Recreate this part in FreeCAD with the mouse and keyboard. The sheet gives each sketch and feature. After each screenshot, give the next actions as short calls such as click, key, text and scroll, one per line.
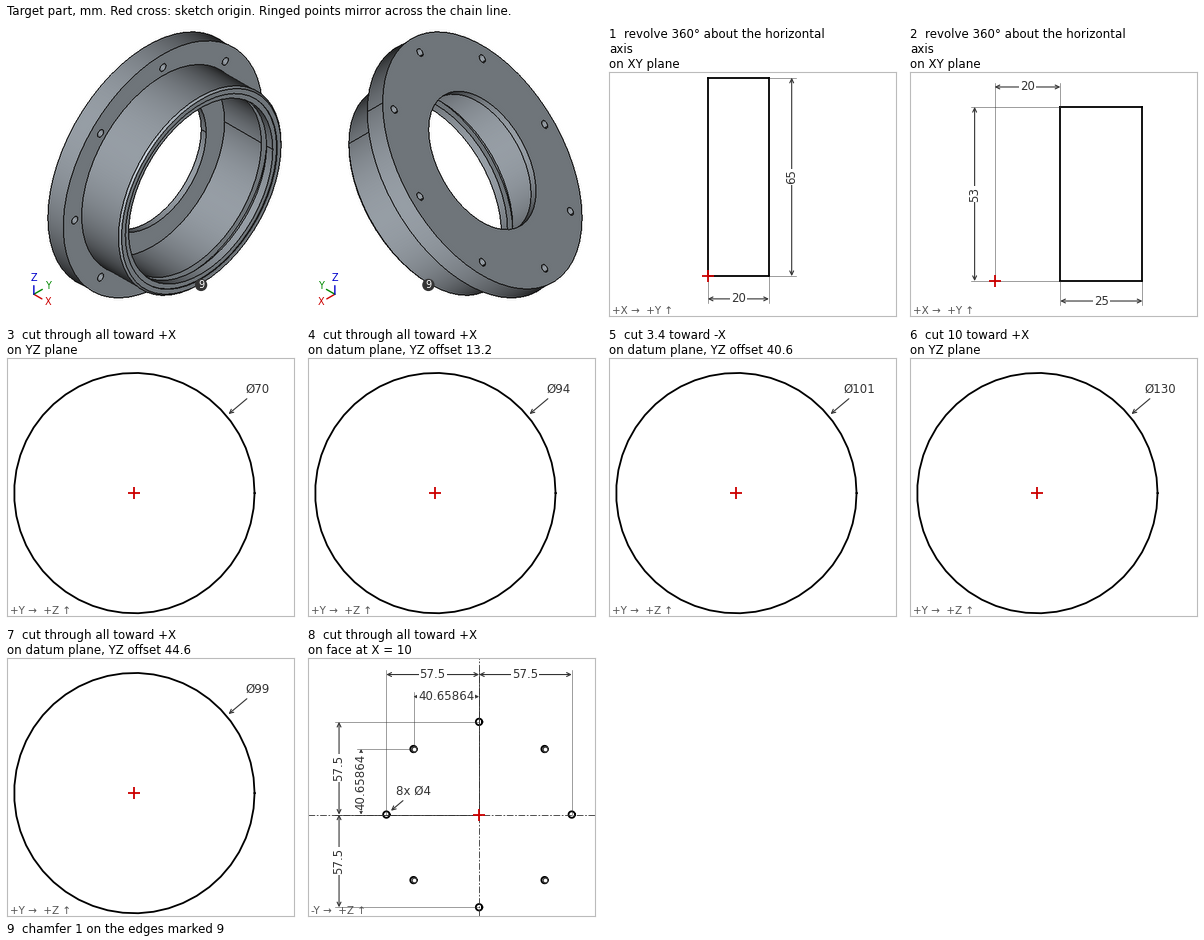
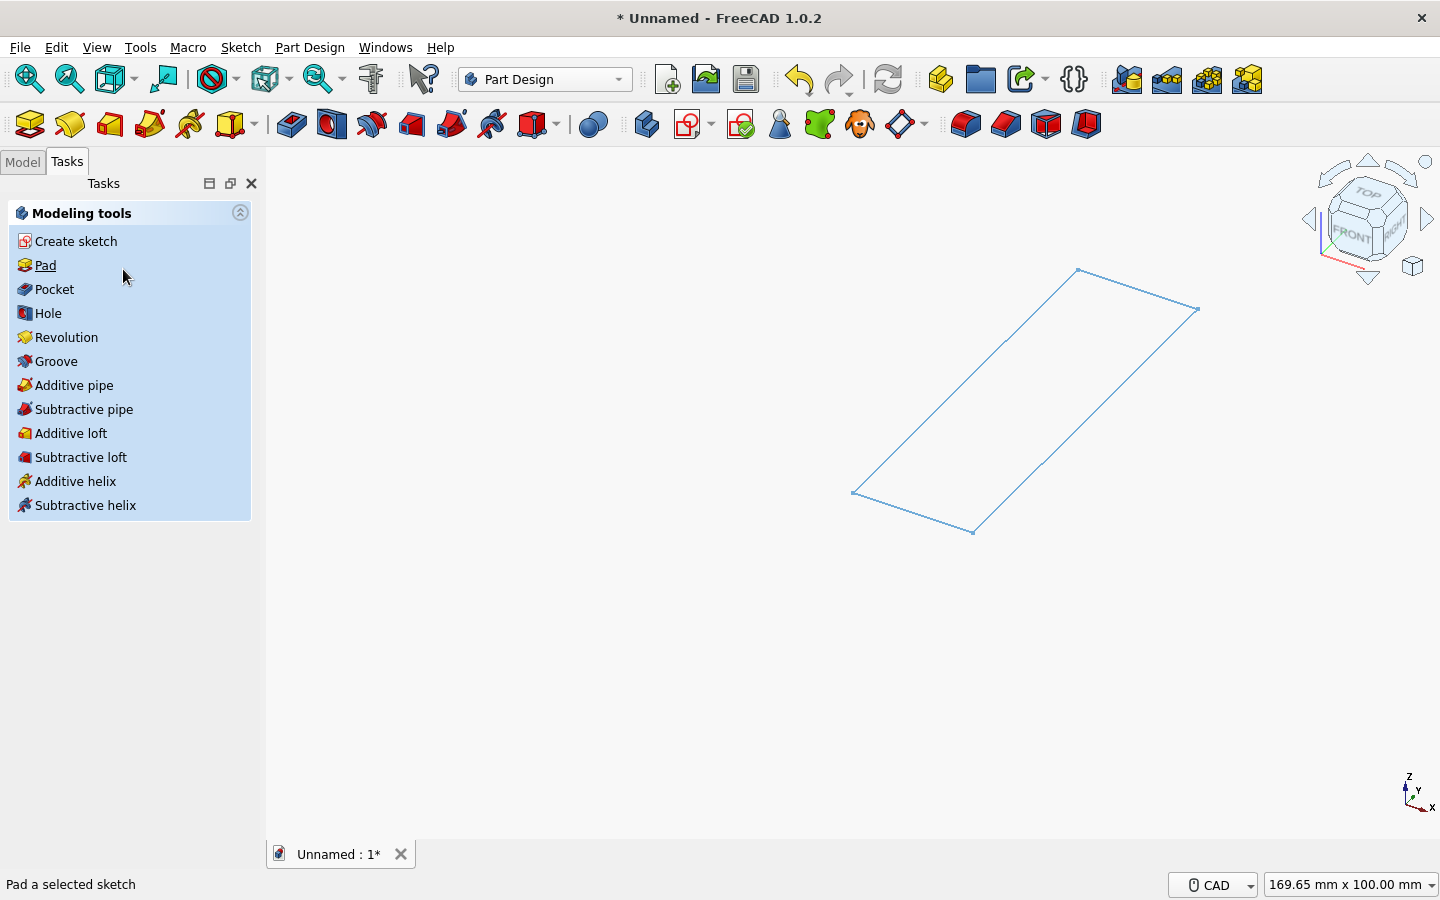
click(70, 124)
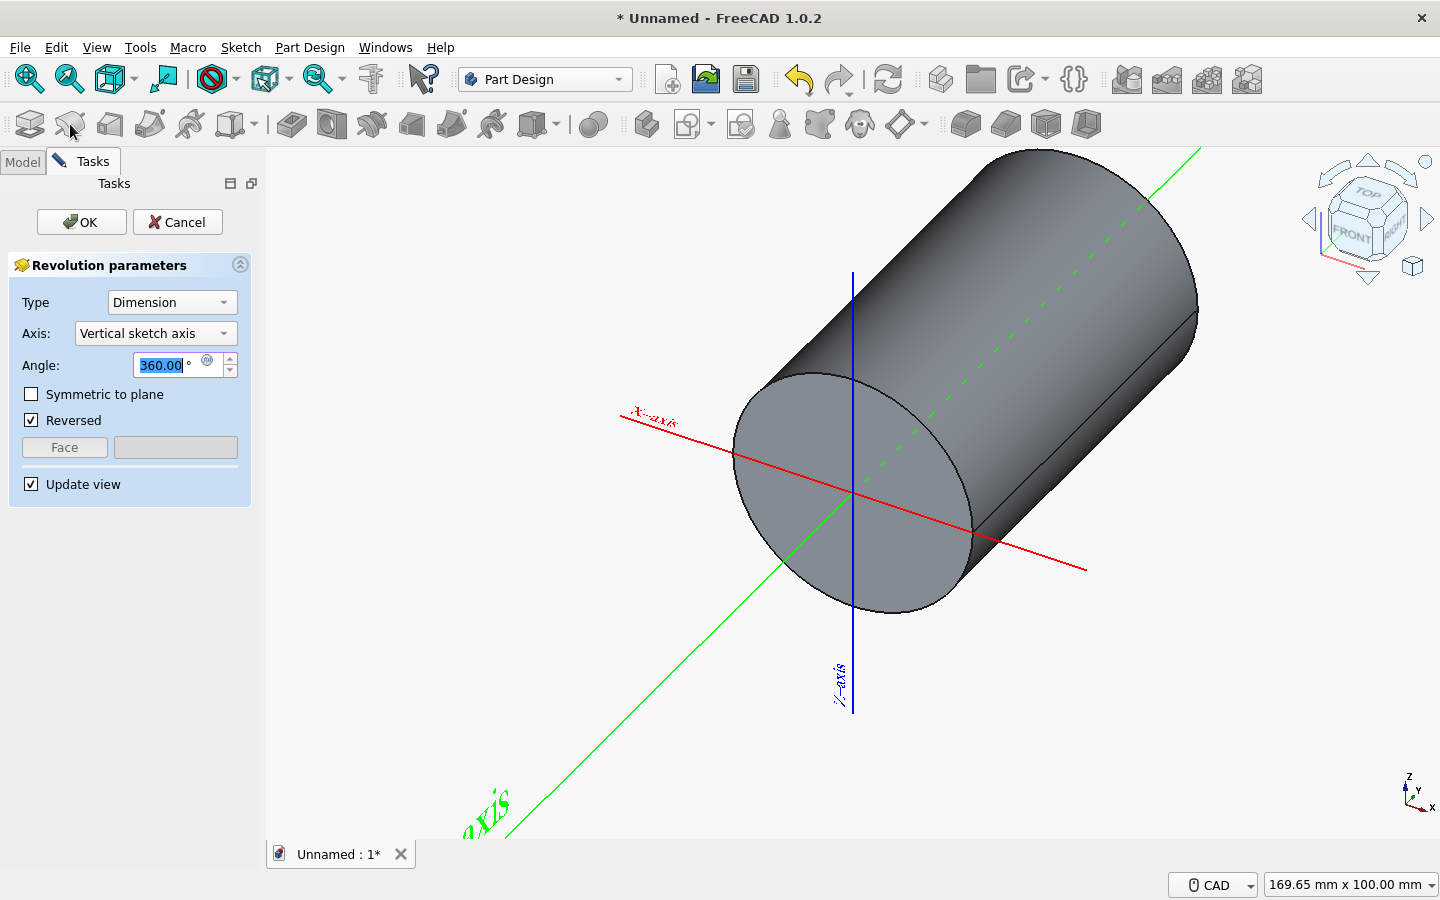
click(156, 334)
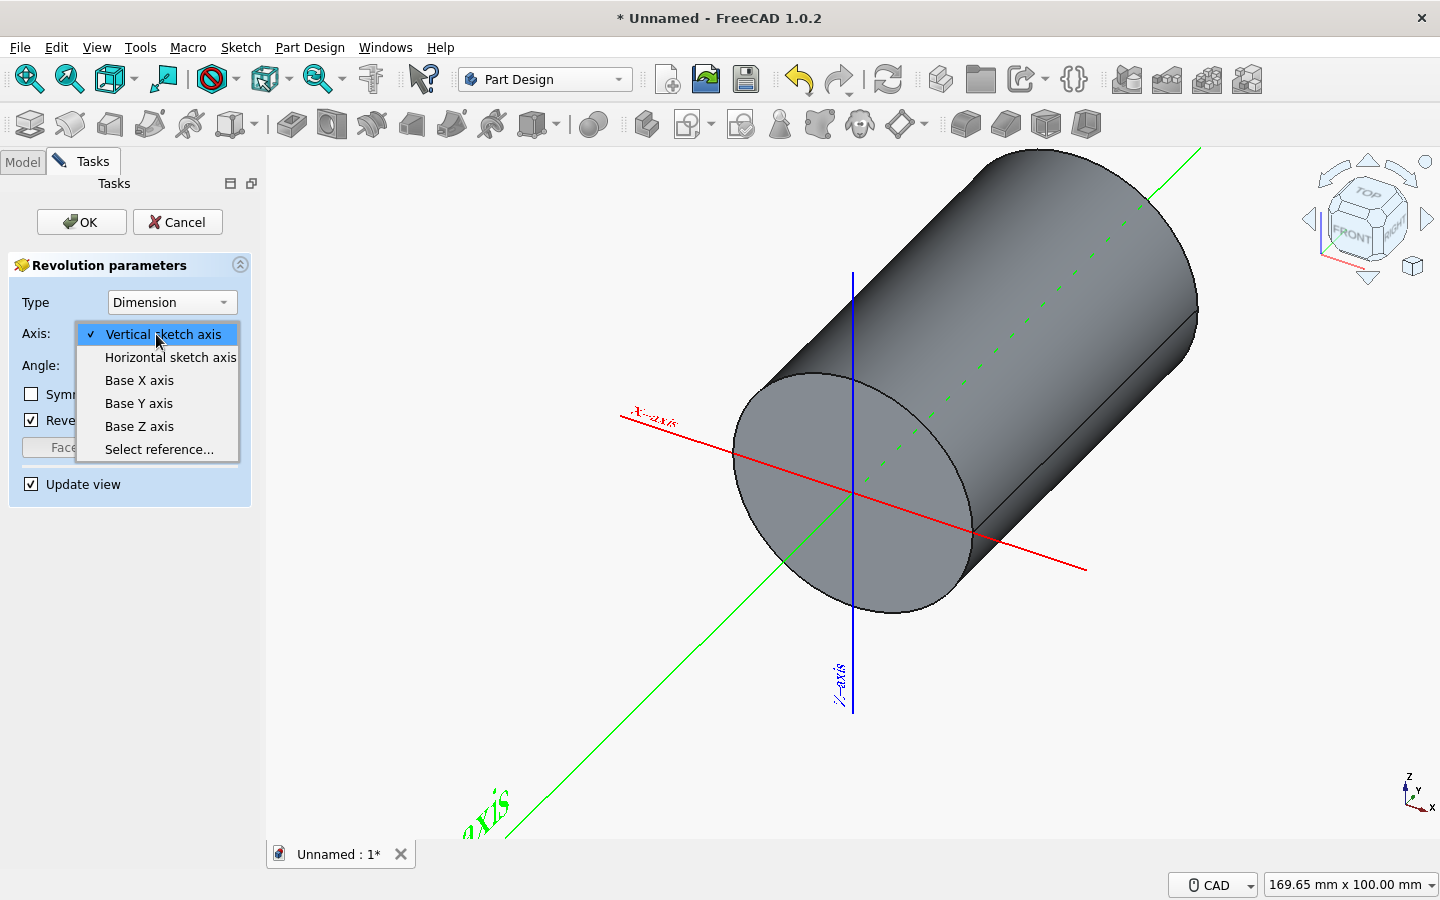
click(156, 358)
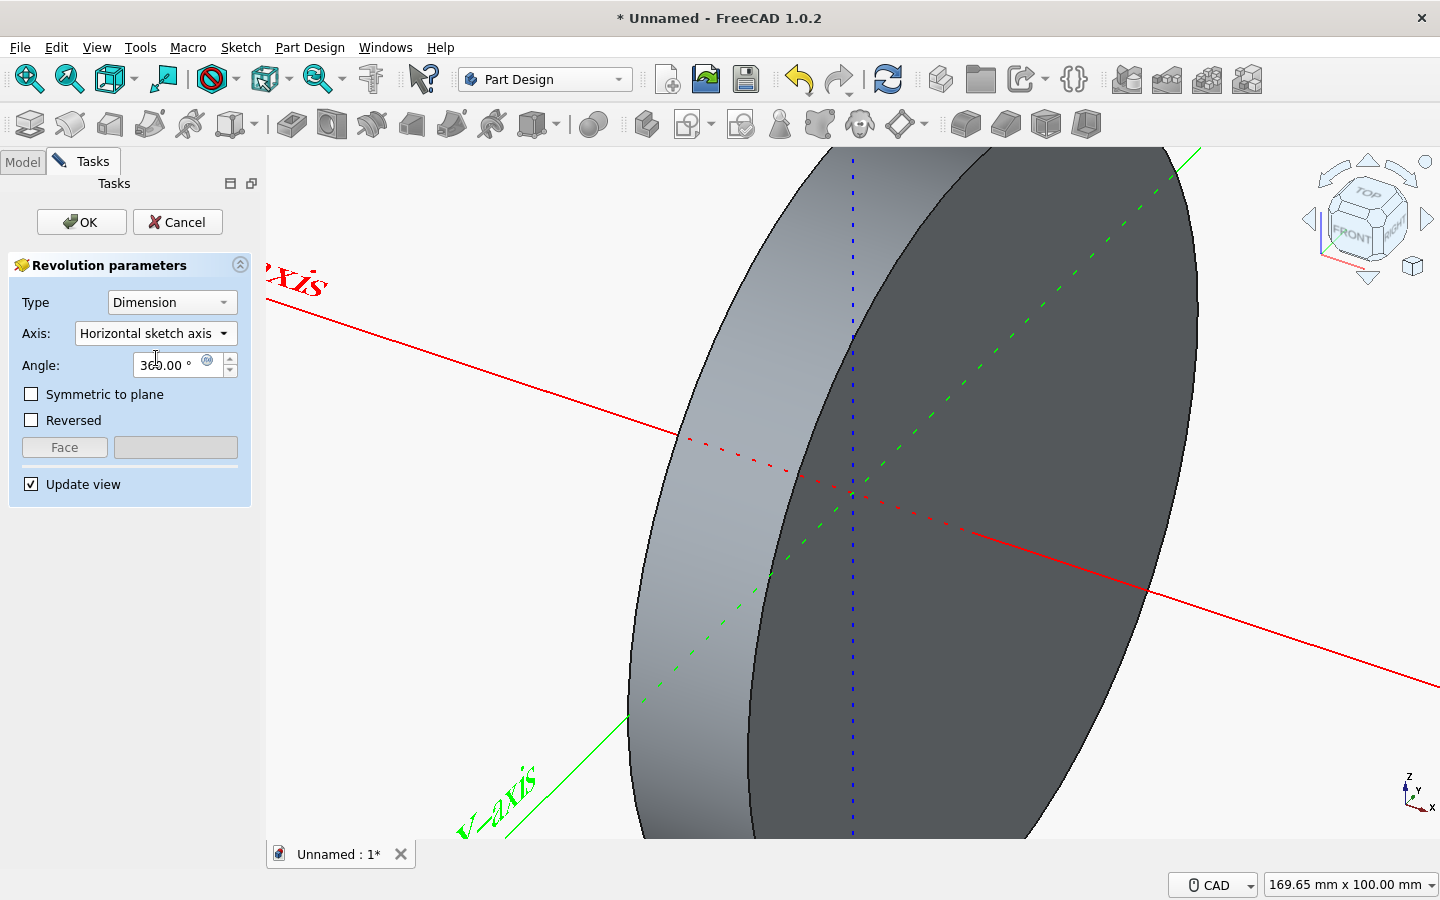
click(82, 222)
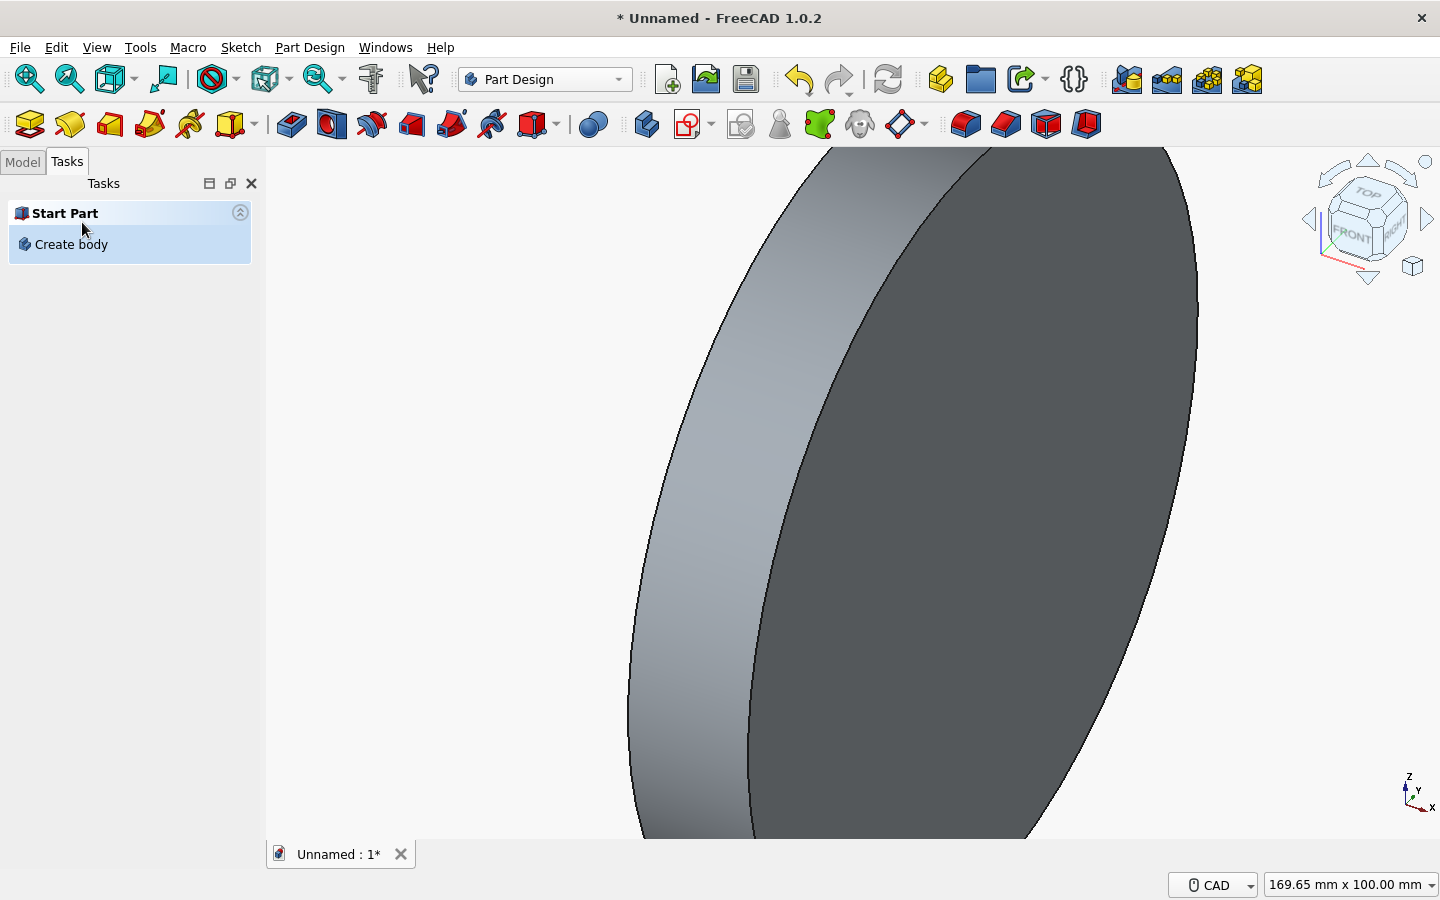
click(30, 80)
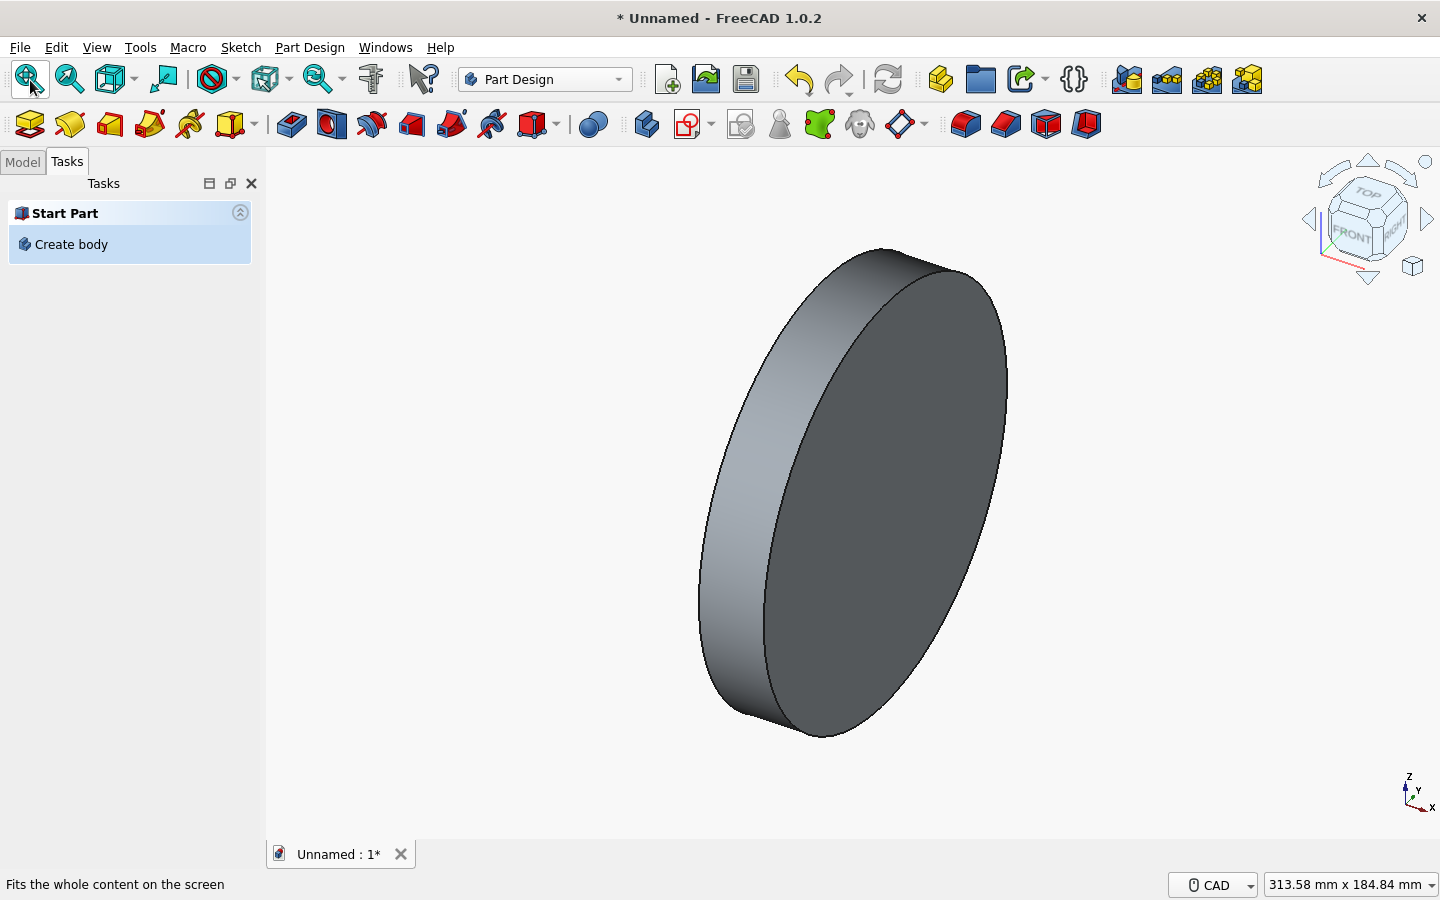
click(688, 124)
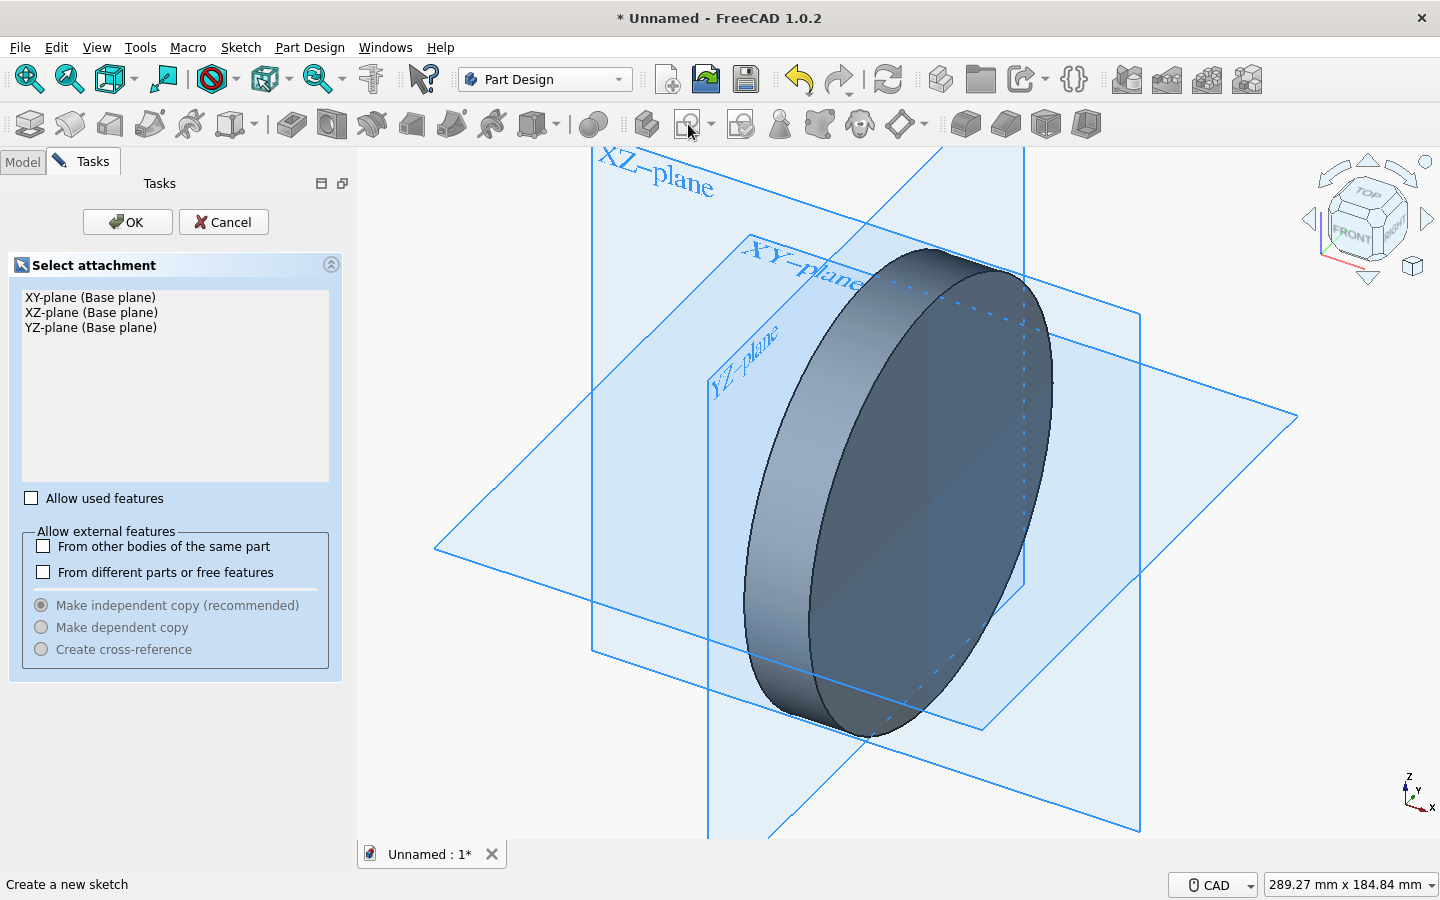
click(82, 298)